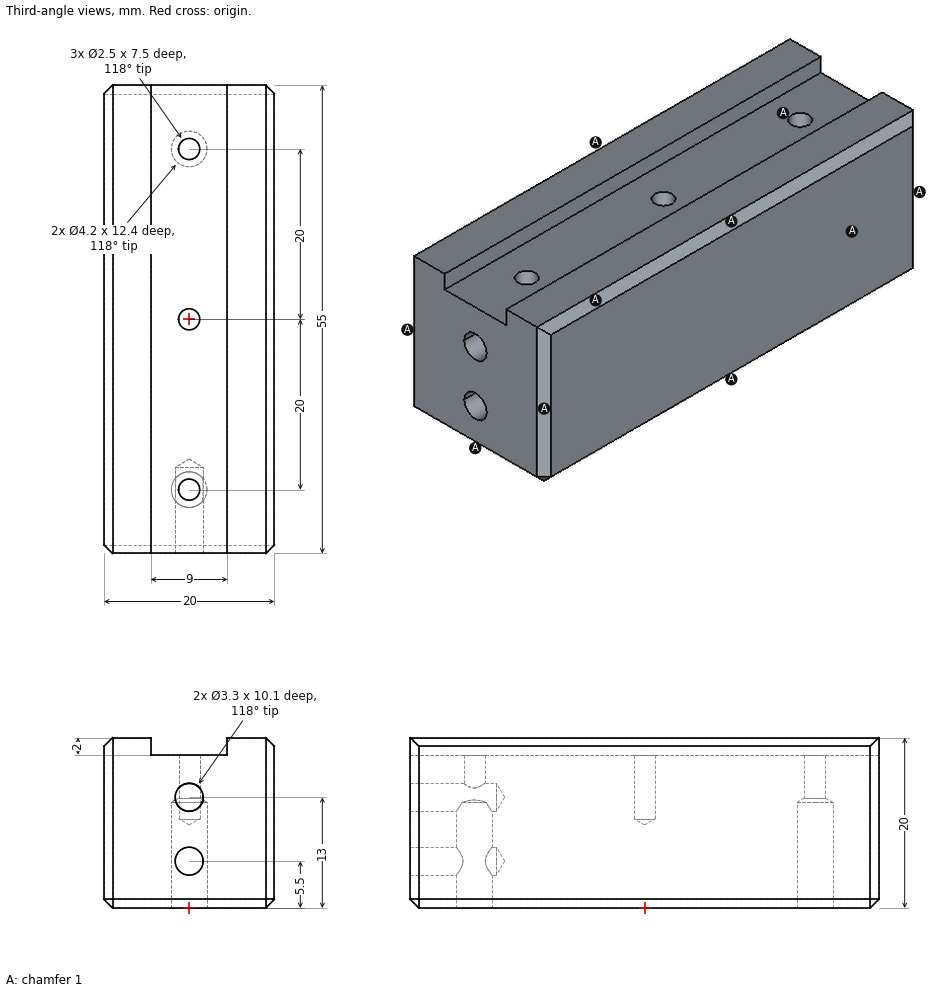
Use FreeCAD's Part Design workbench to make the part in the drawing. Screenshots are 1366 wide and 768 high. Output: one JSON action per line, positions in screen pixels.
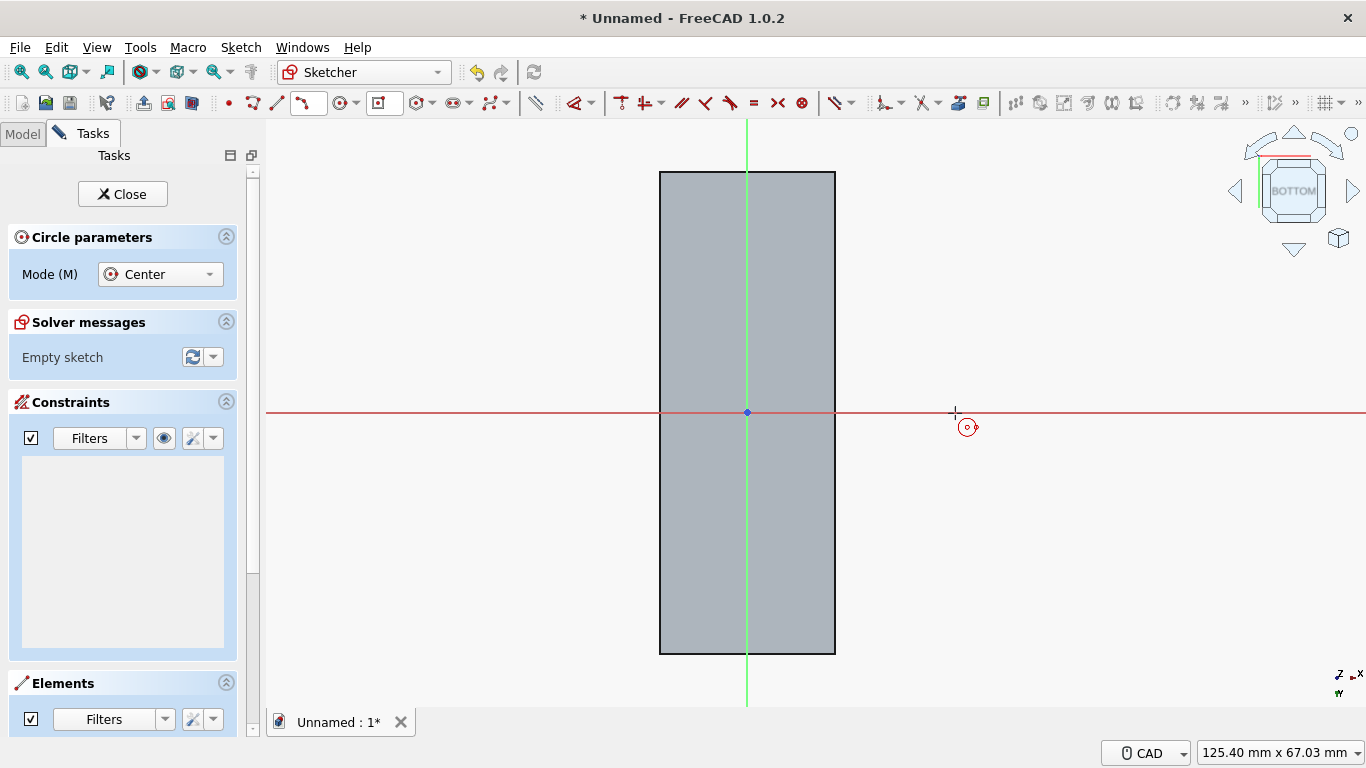
{"action": "scroll", "coordinate": [747, 588], "scroll_direction": "up", "scroll_amount": 2}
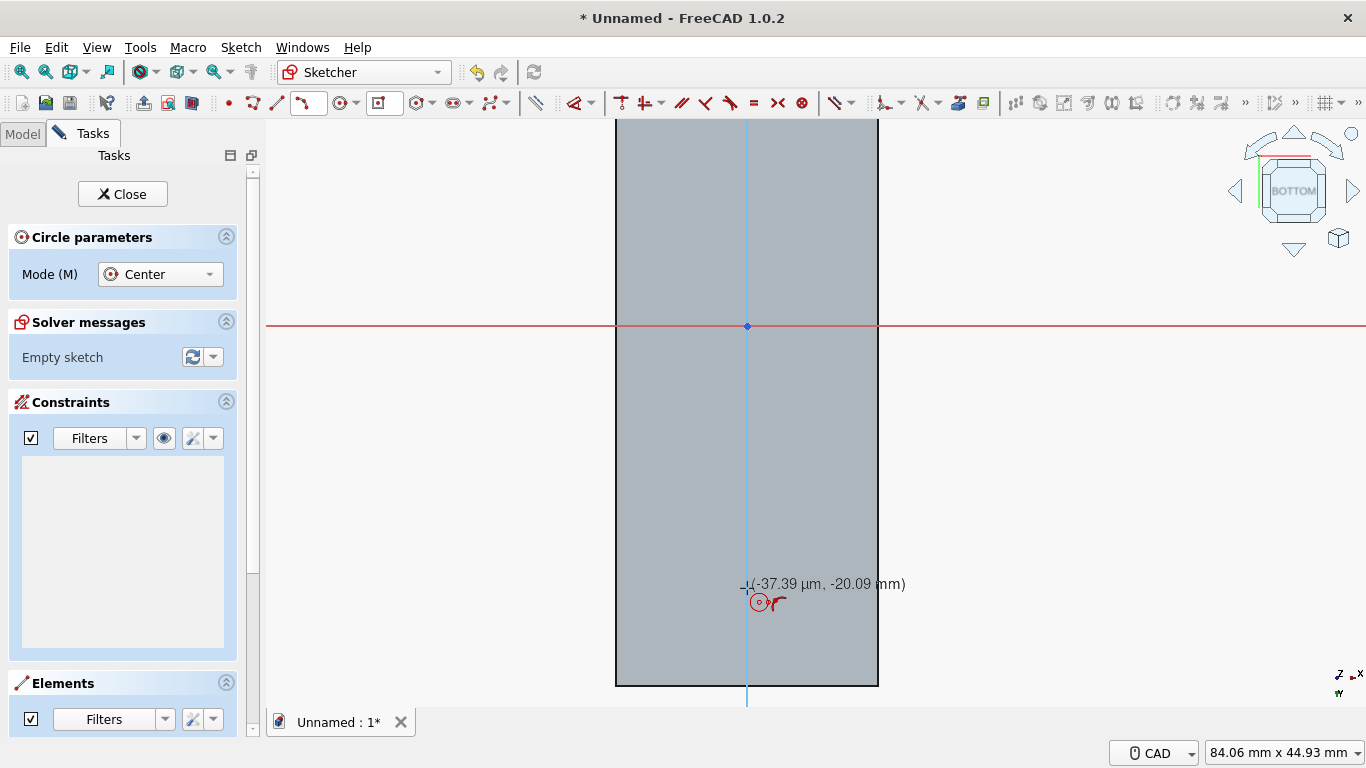
{"action": "left_click", "coordinate": [747, 588]}
{"action": "mouse_move", "coordinate": [767, 568]}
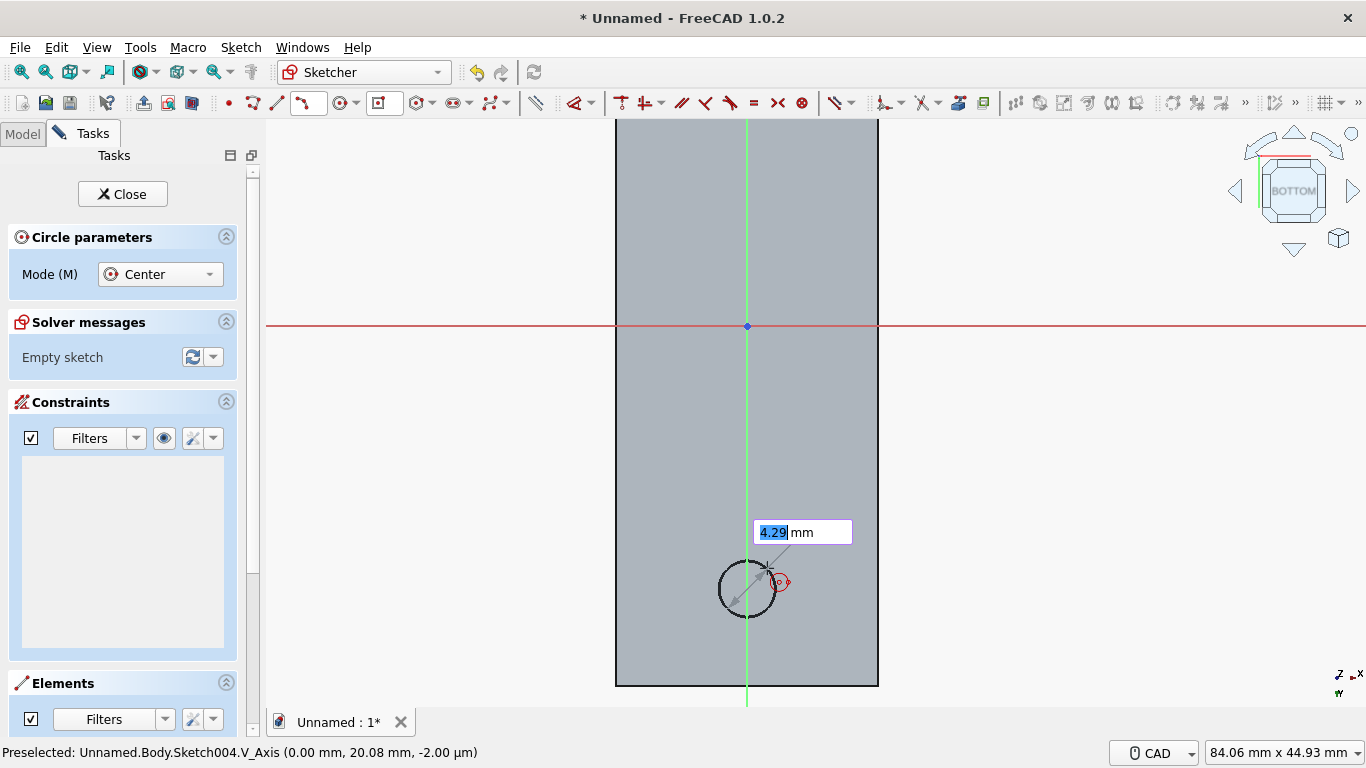
{"action": "type", "text": "4.2"}
{"action": "key", "text": "Return"}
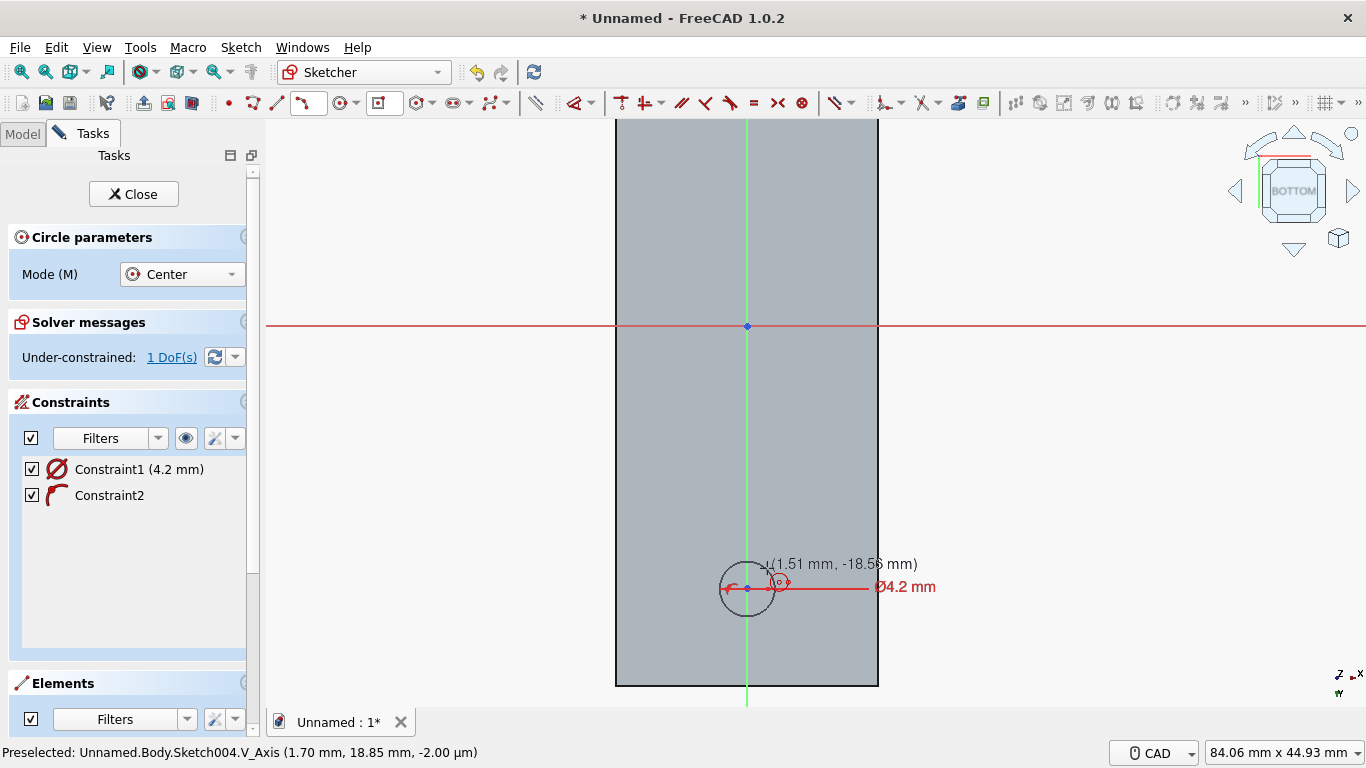
{"action": "scroll", "coordinate": [748, 590], "scroll_direction": "down", "scroll_amount": 2}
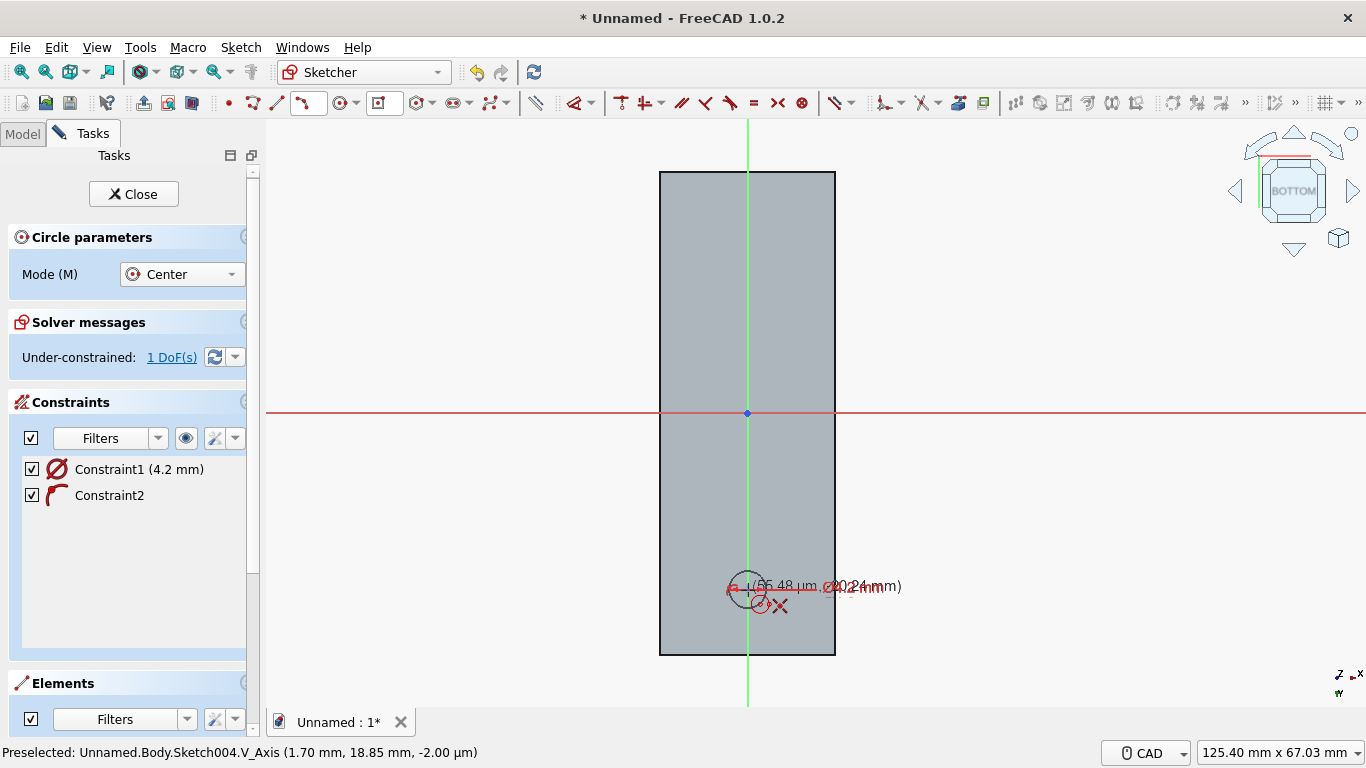
{"action": "scroll", "coordinate": [748, 238], "scroll_direction": "up", "scroll_amount": 2}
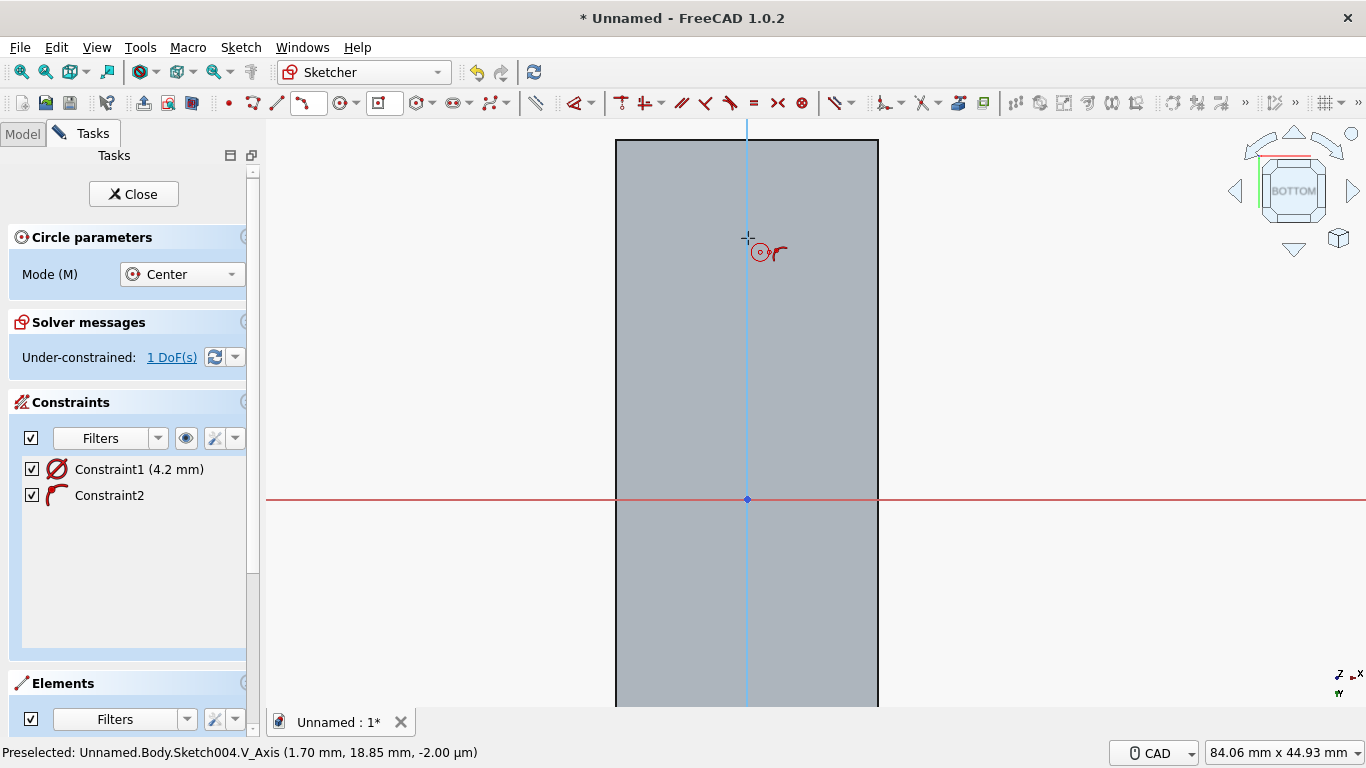
{"action": "left_click", "coordinate": [747, 238]}
{"action": "mouse_move", "coordinate": [767, 218]}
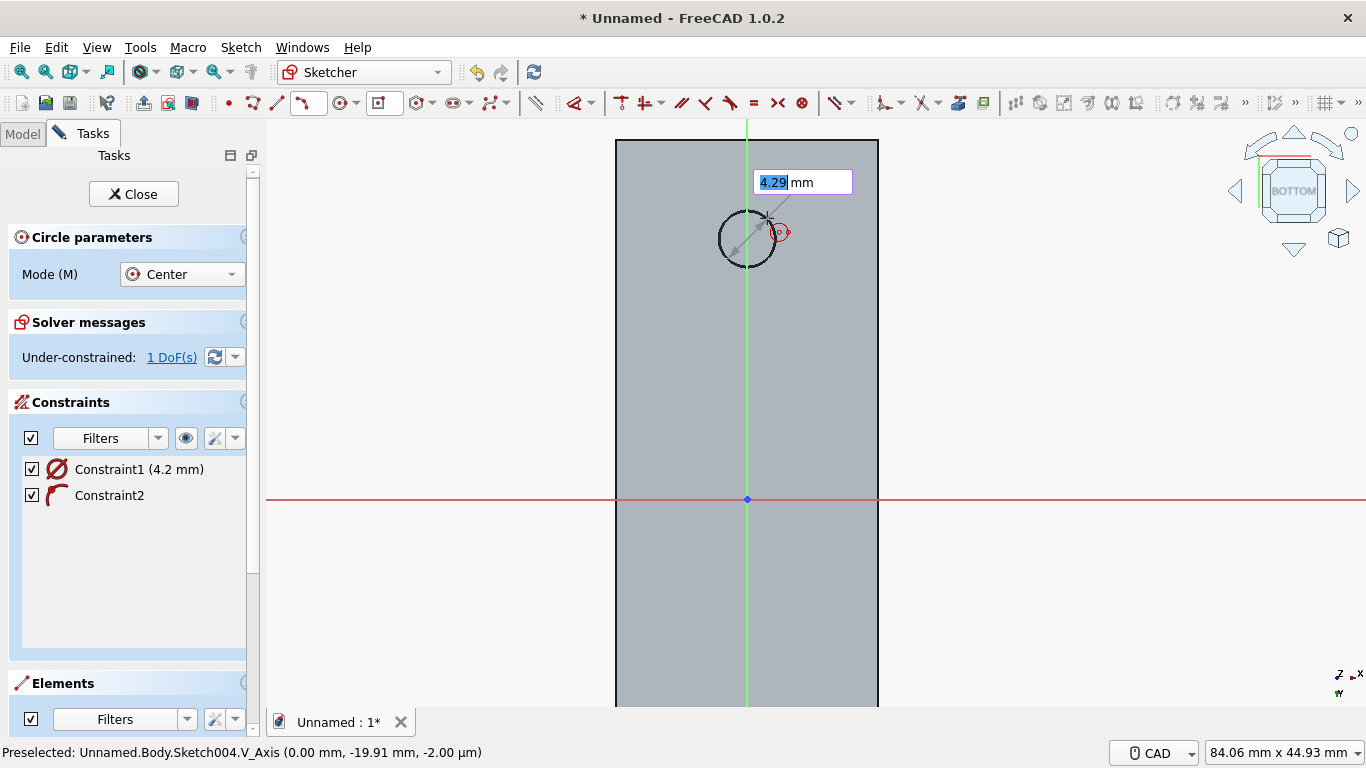
{"action": "type", "text": "4.2"}
{"action": "key", "text": "Return"}
{"action": "key", "text": "Escape"}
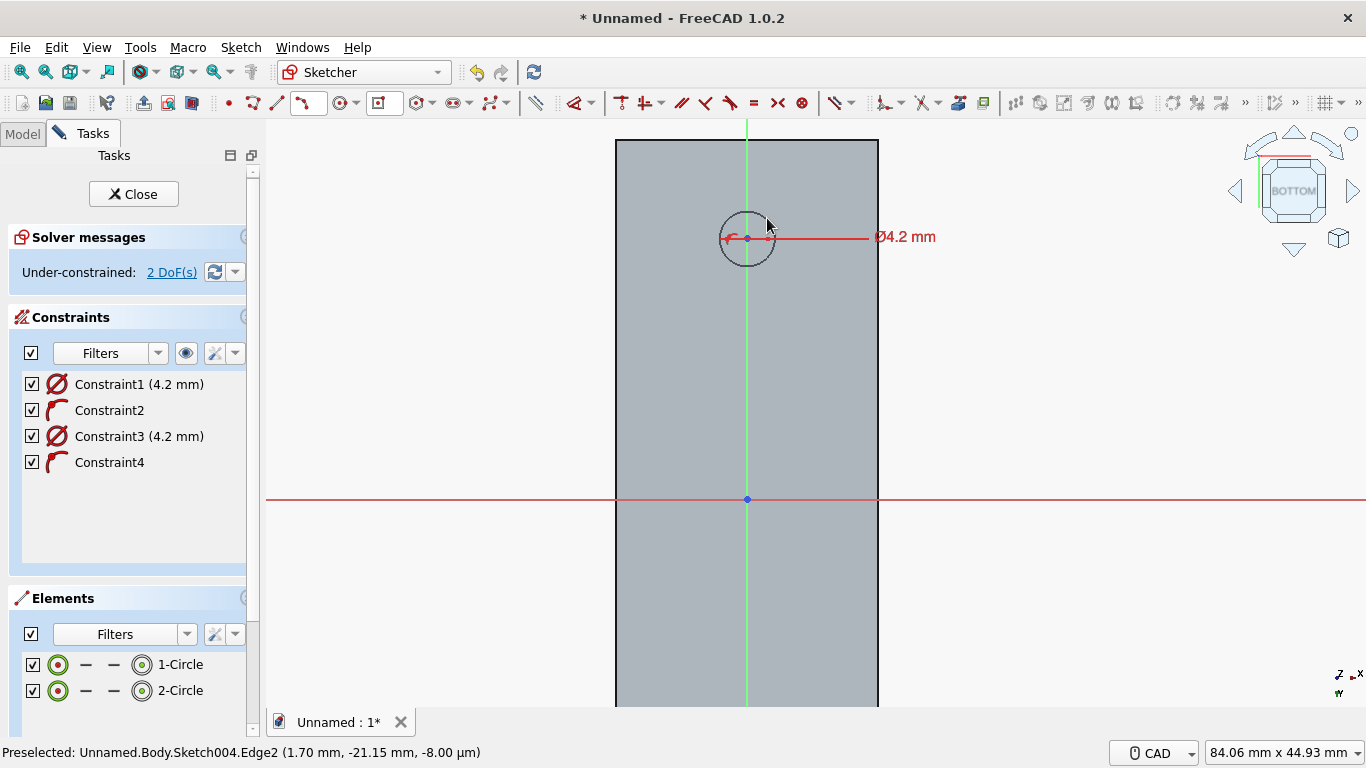
{"action": "key", "text": "d"}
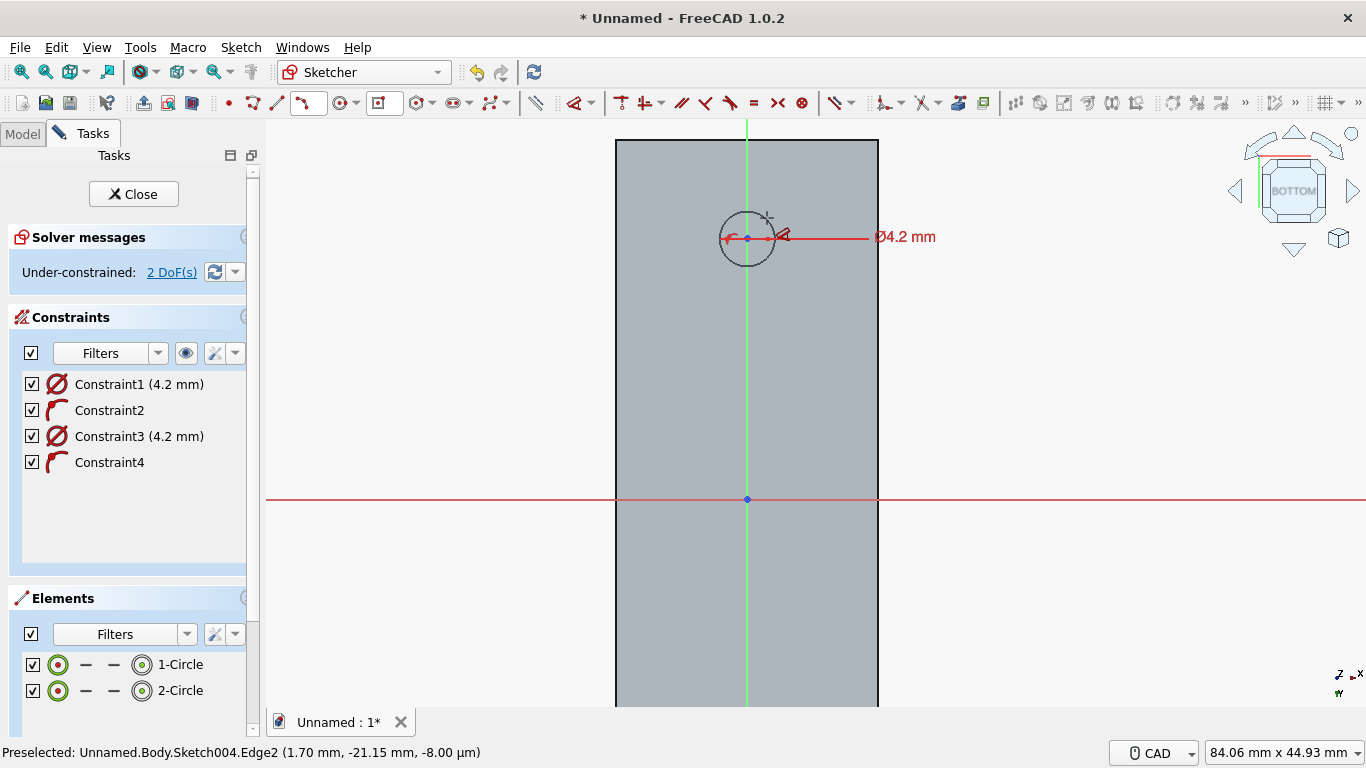
{"action": "scroll", "coordinate": [748, 237], "scroll_direction": "down", "scroll_amount": 2}